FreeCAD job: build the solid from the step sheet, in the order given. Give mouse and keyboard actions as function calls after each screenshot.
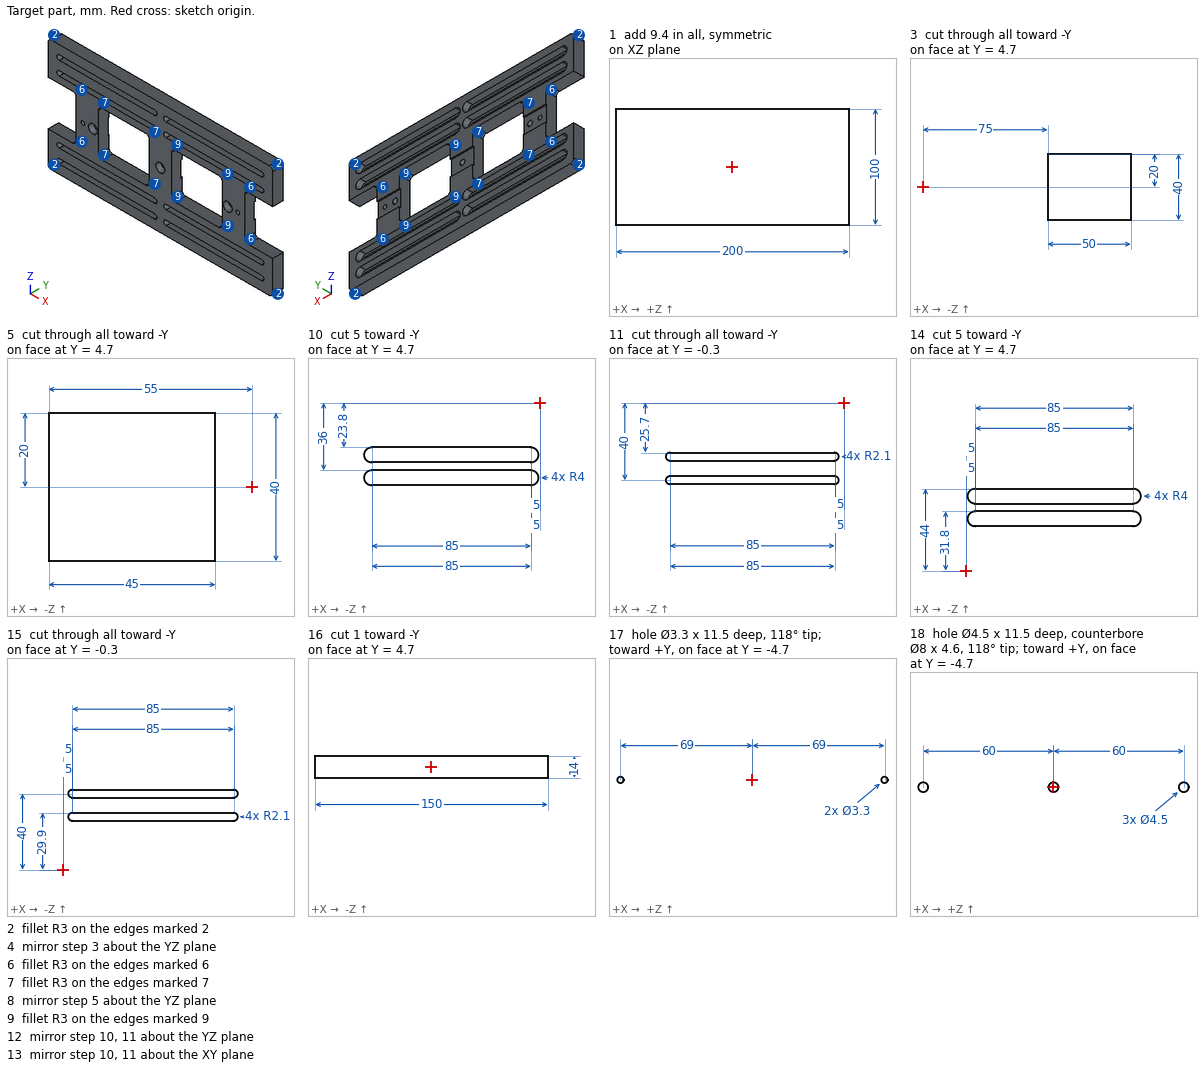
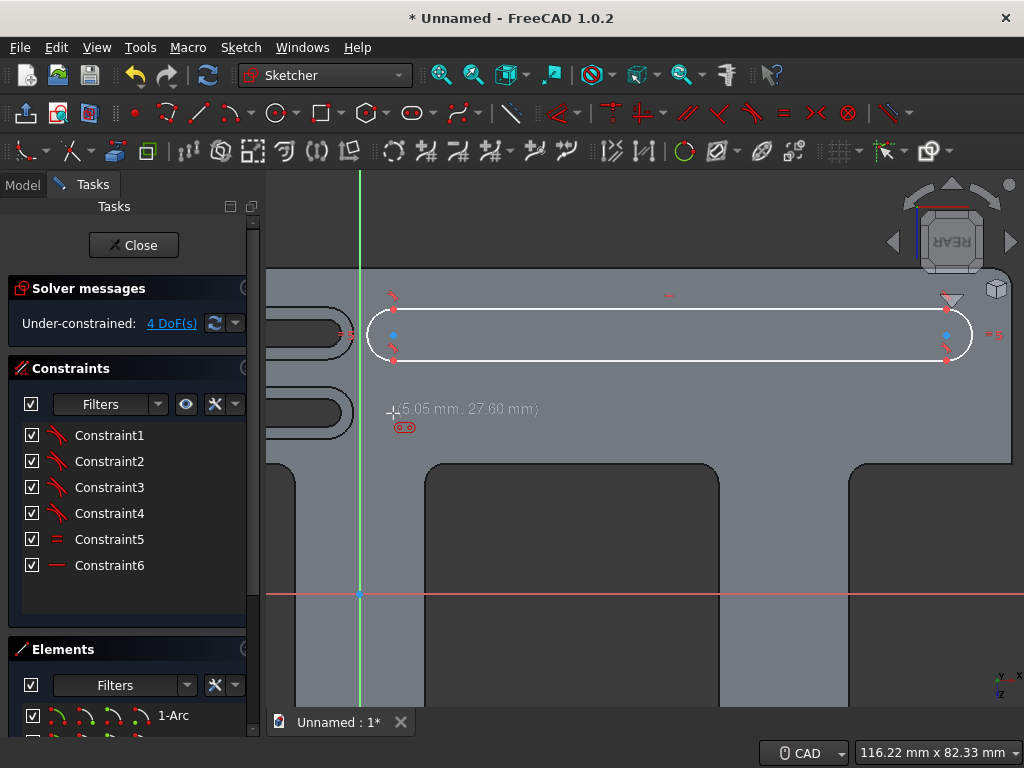
click(393, 413)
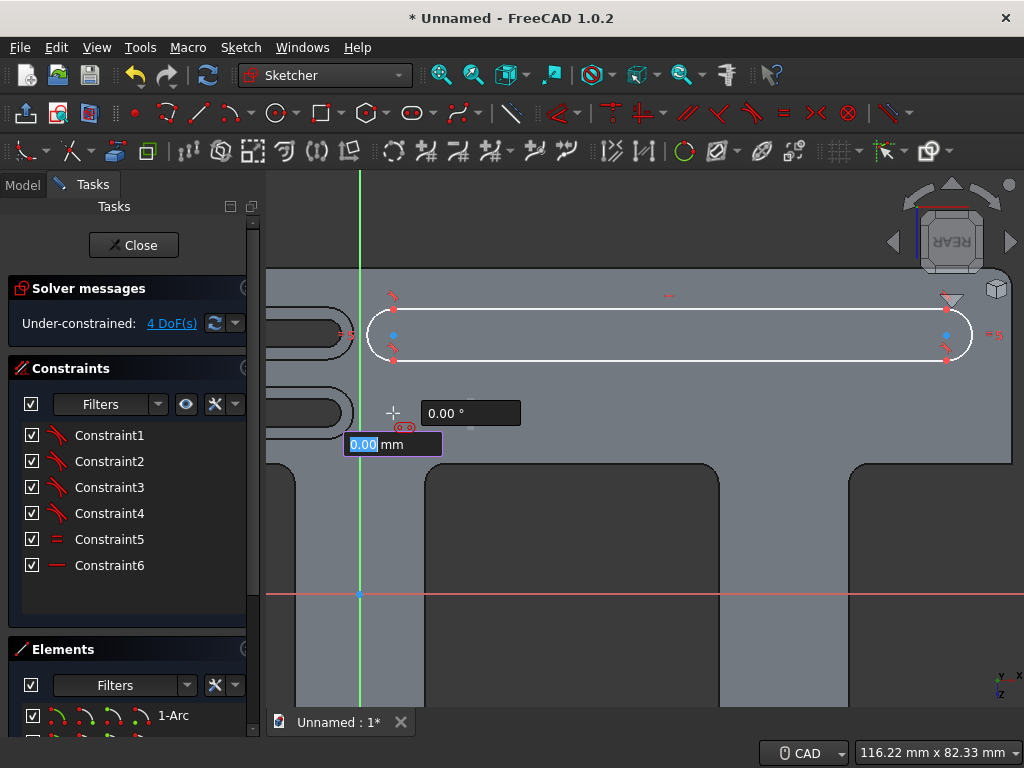
scroll(393, 413, down, 2)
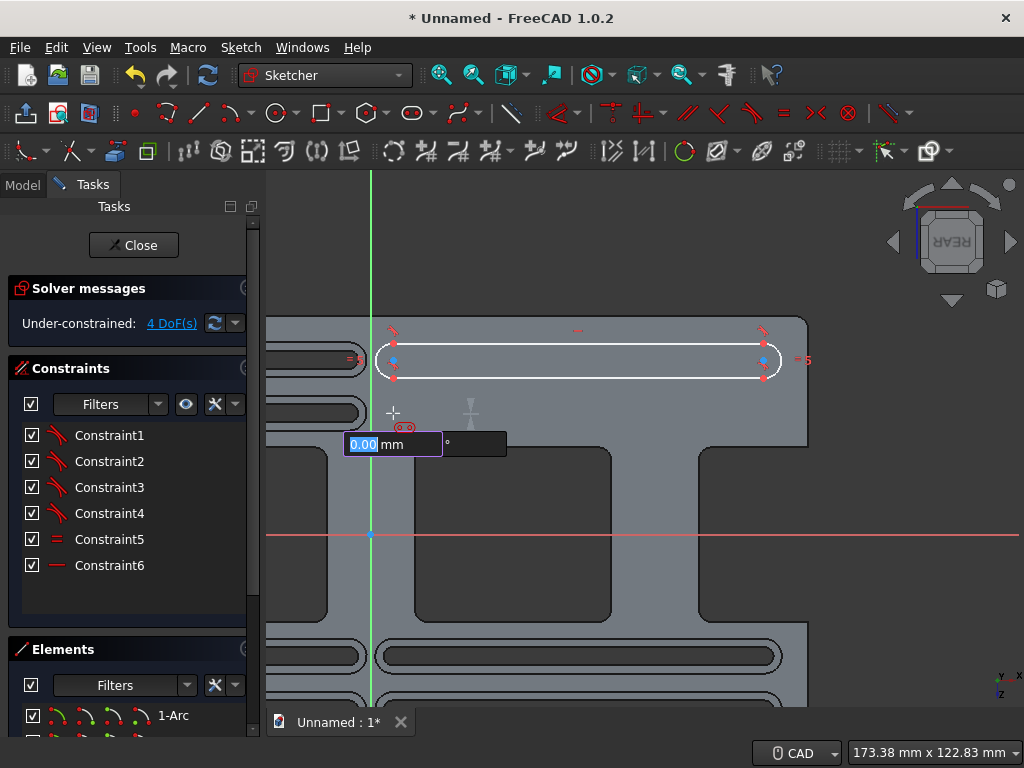
click(764, 413)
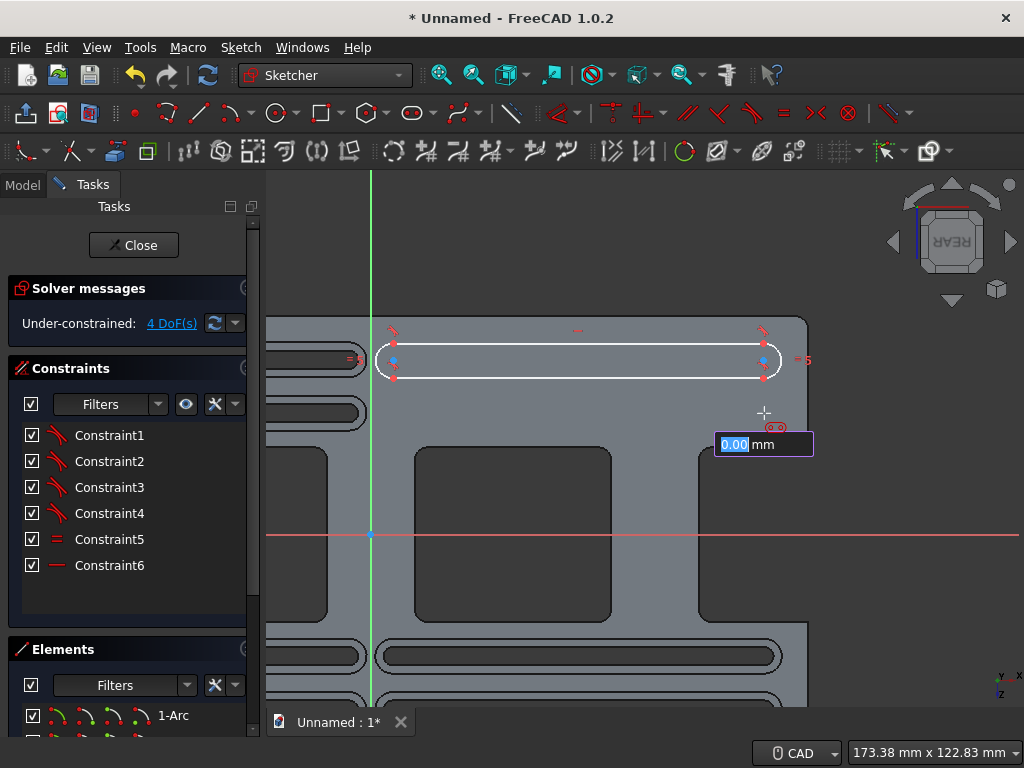
click(579, 396)
key(Escape)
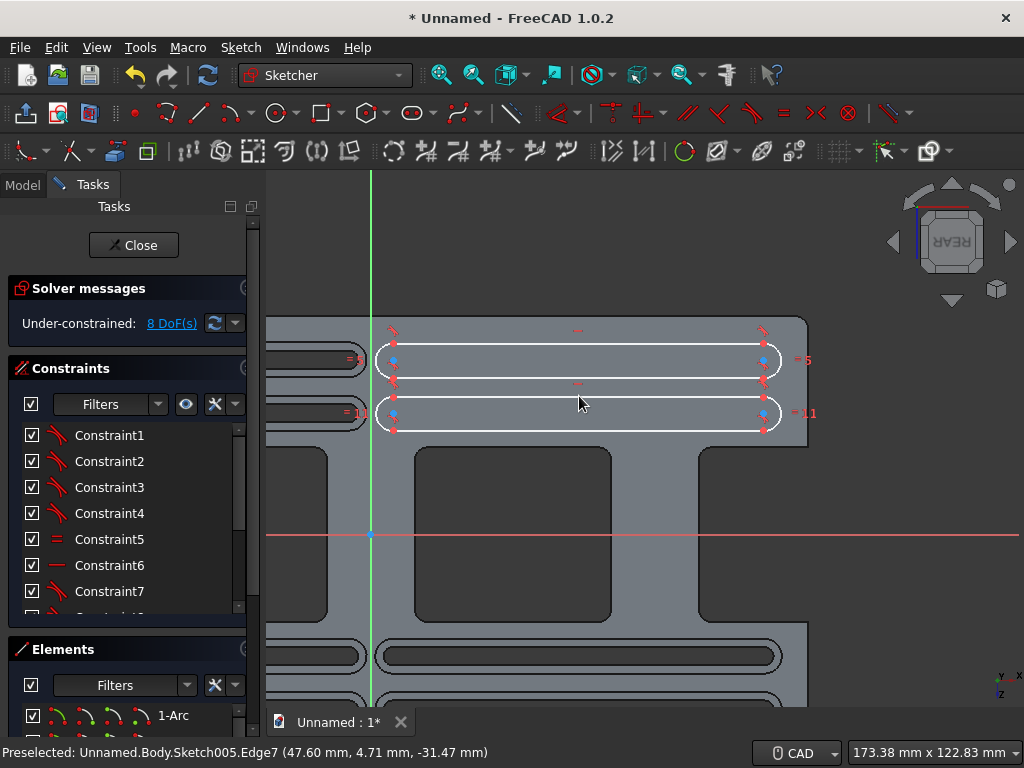
scroll(383, 347, up, 2)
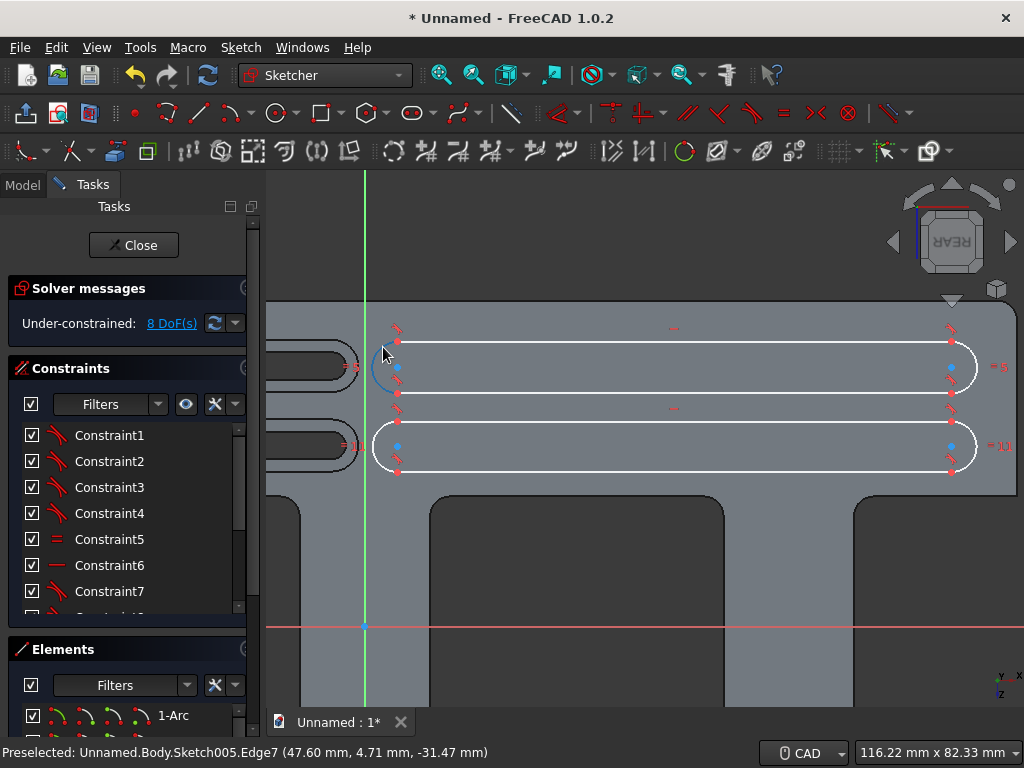
click(383, 347)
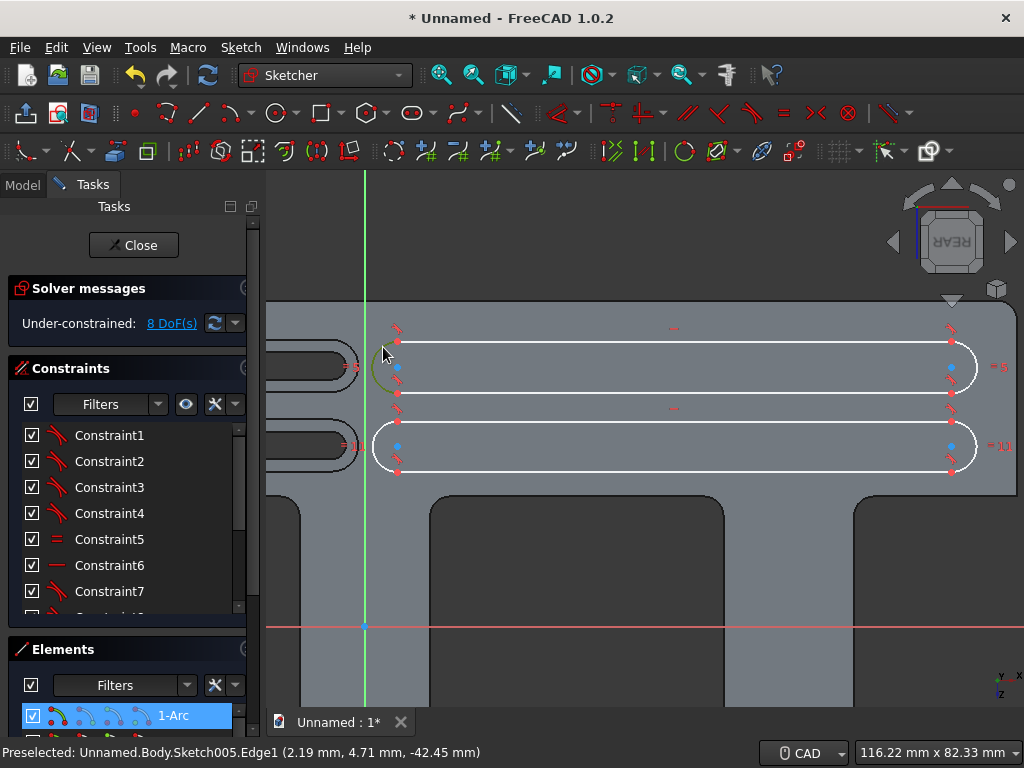
click(378, 432)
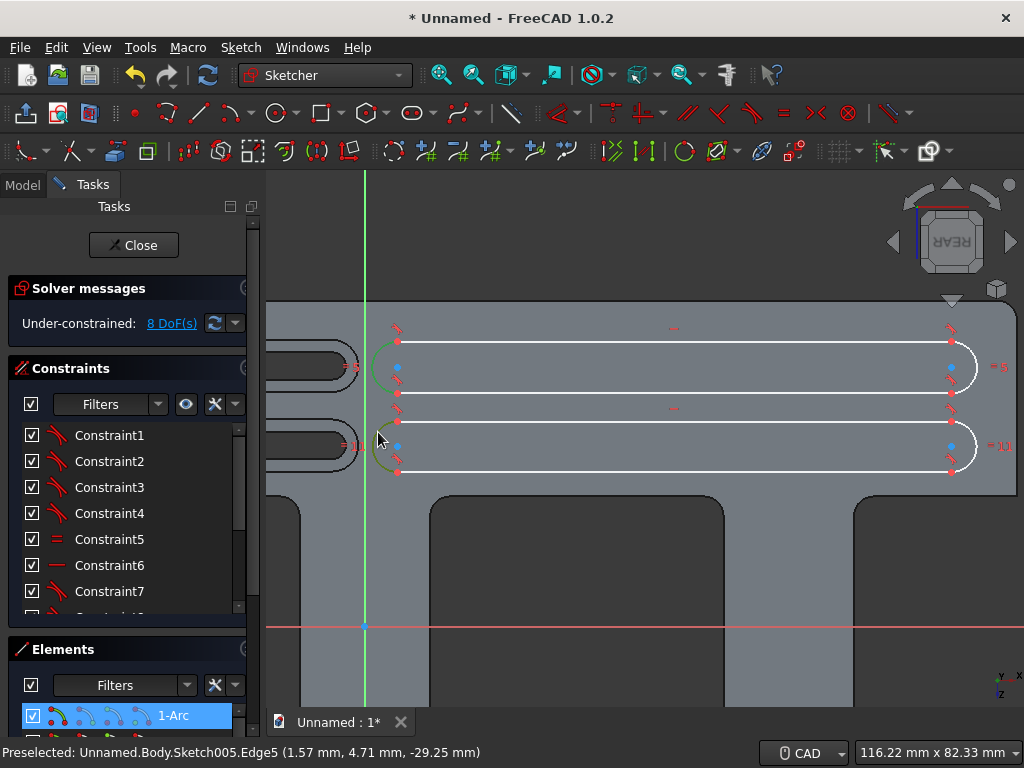
click(784, 114)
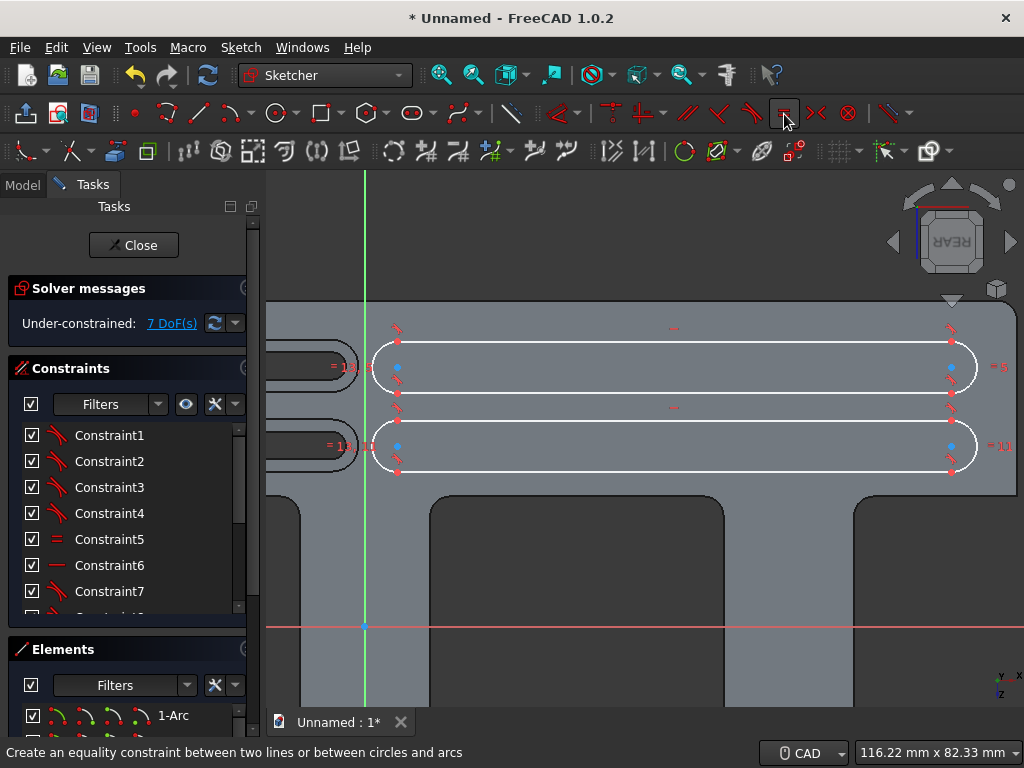
key(d)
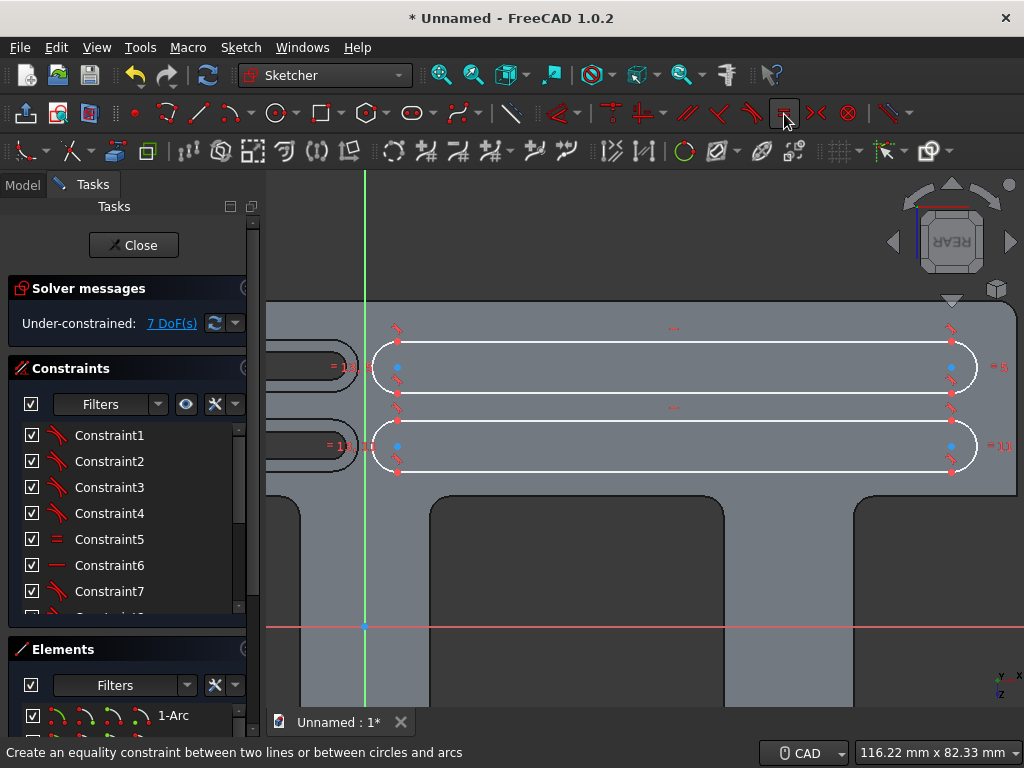
scroll(377, 352, up, 3)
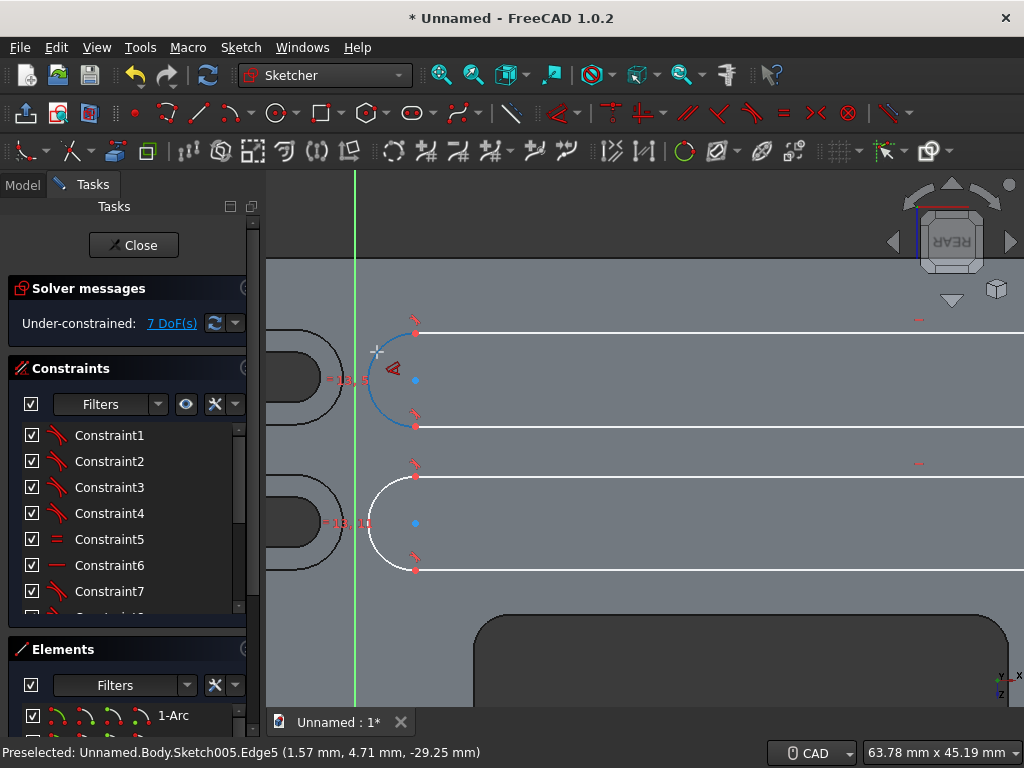
click(377, 353)
click(381, 309)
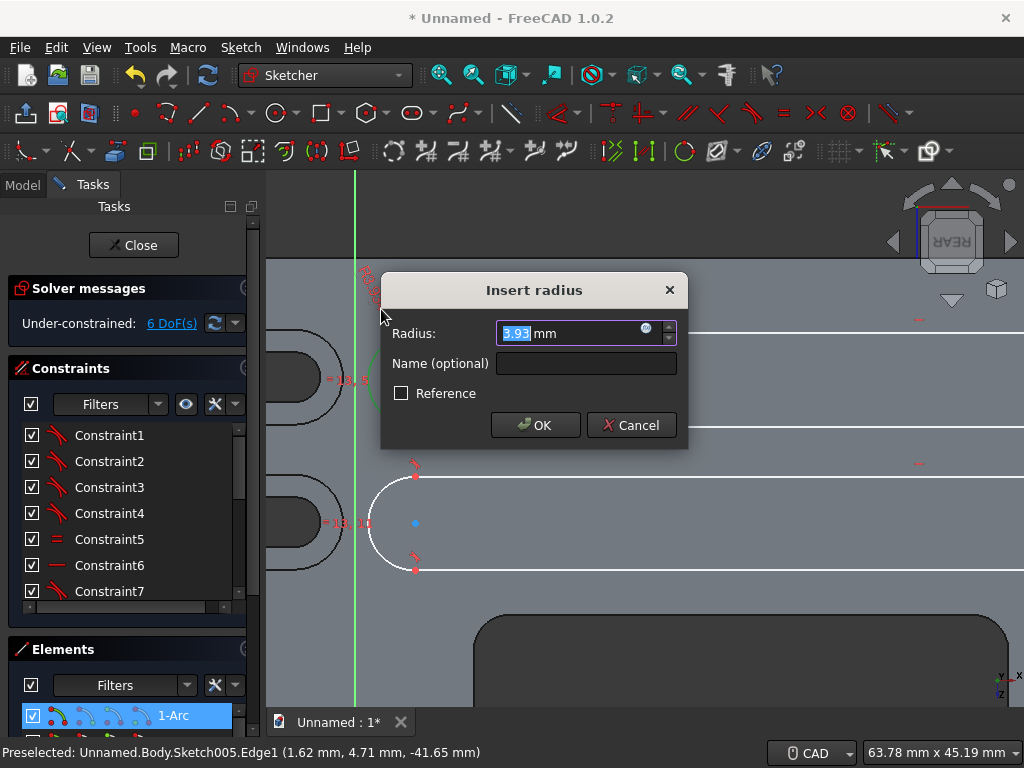
text(4)
key(Return)